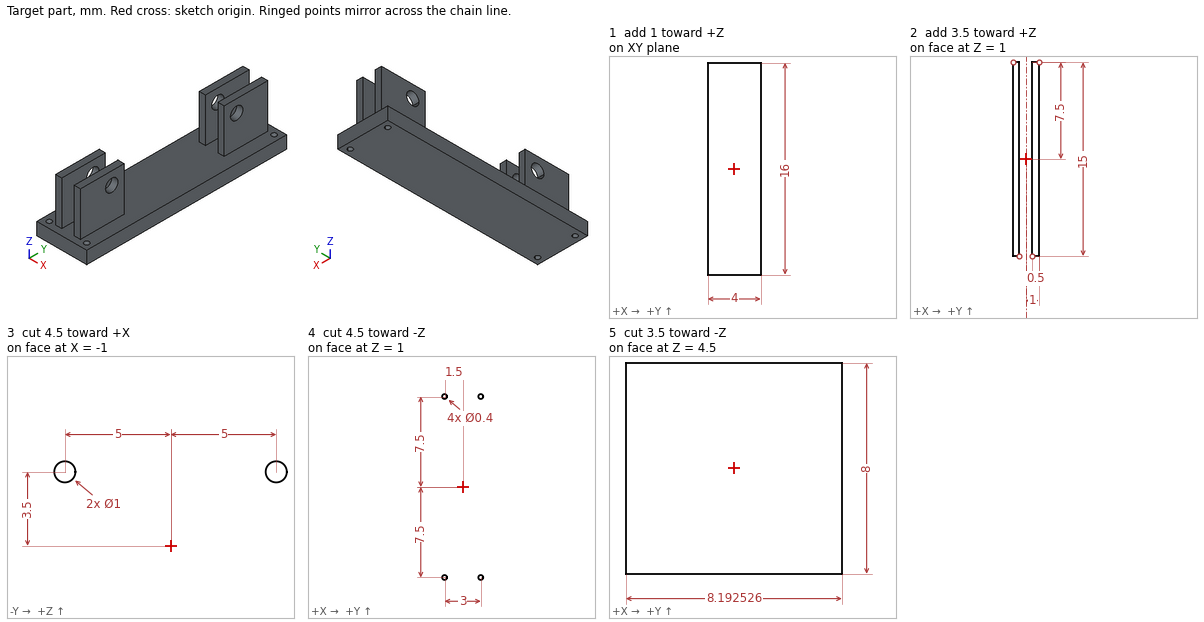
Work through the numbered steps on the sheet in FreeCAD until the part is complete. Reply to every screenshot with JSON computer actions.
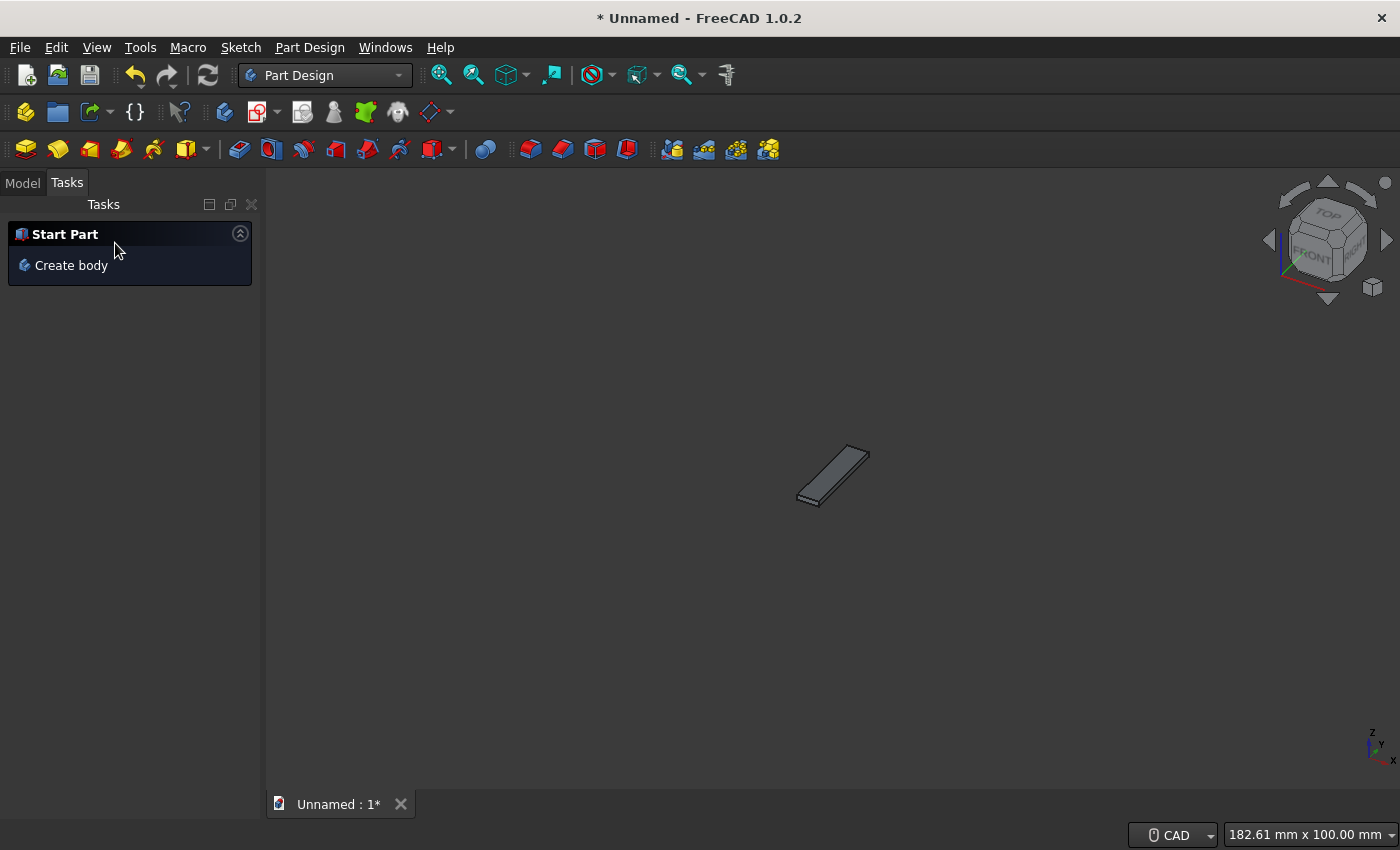
{"action": "key", "text": "v f"}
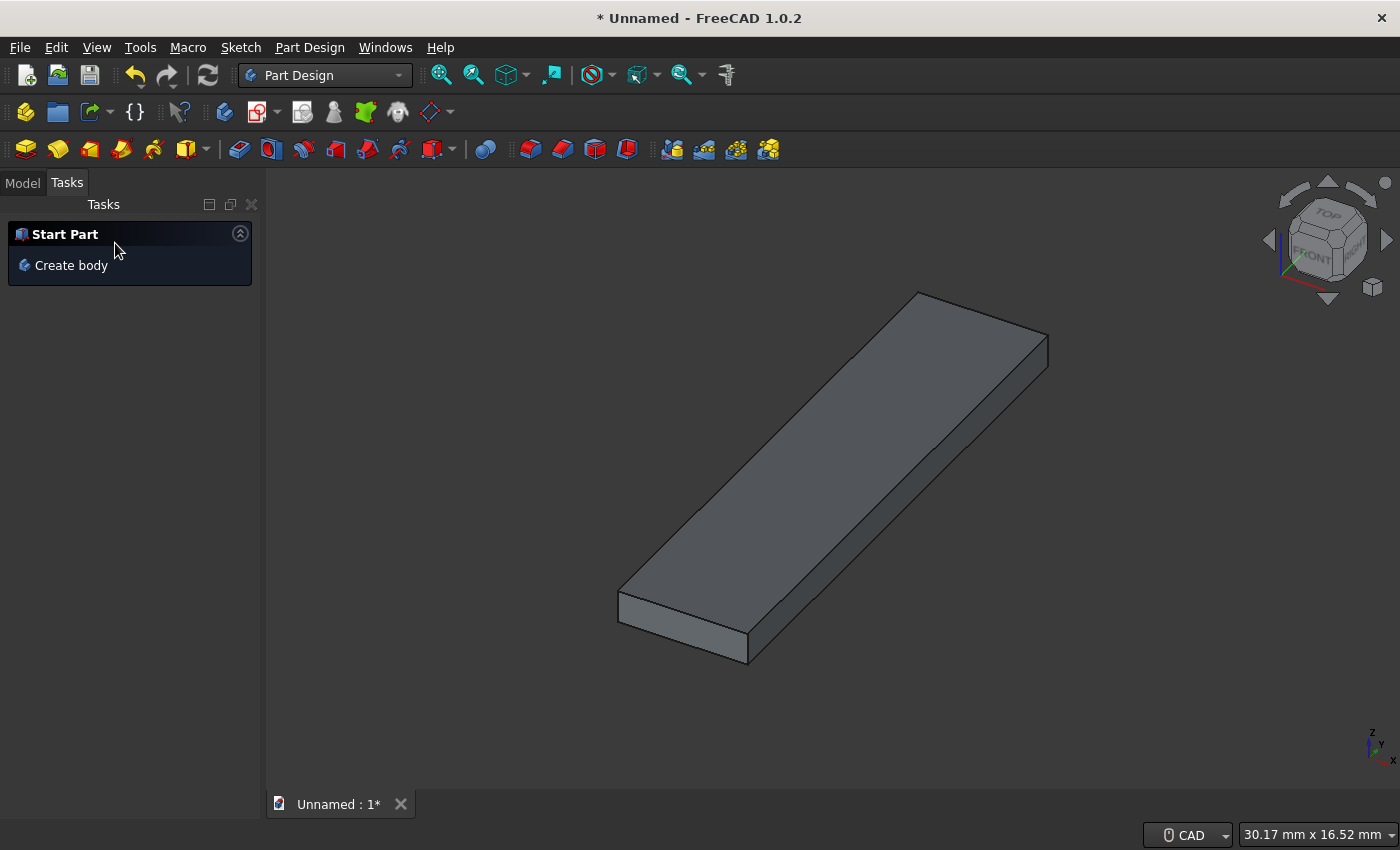
{"action": "left_click", "coordinate": [919, 377]}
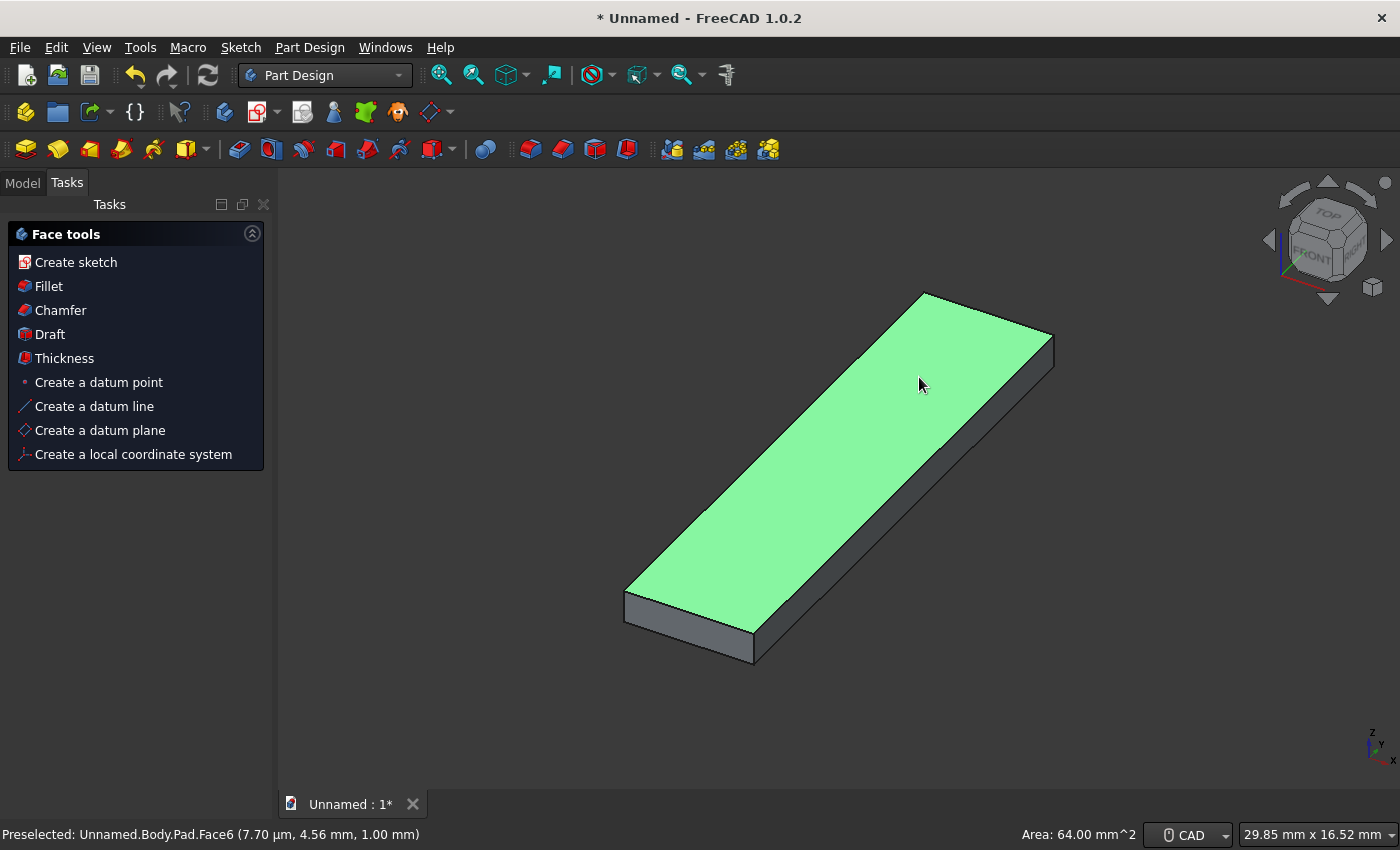
{"action": "left_click", "coordinate": [258, 112]}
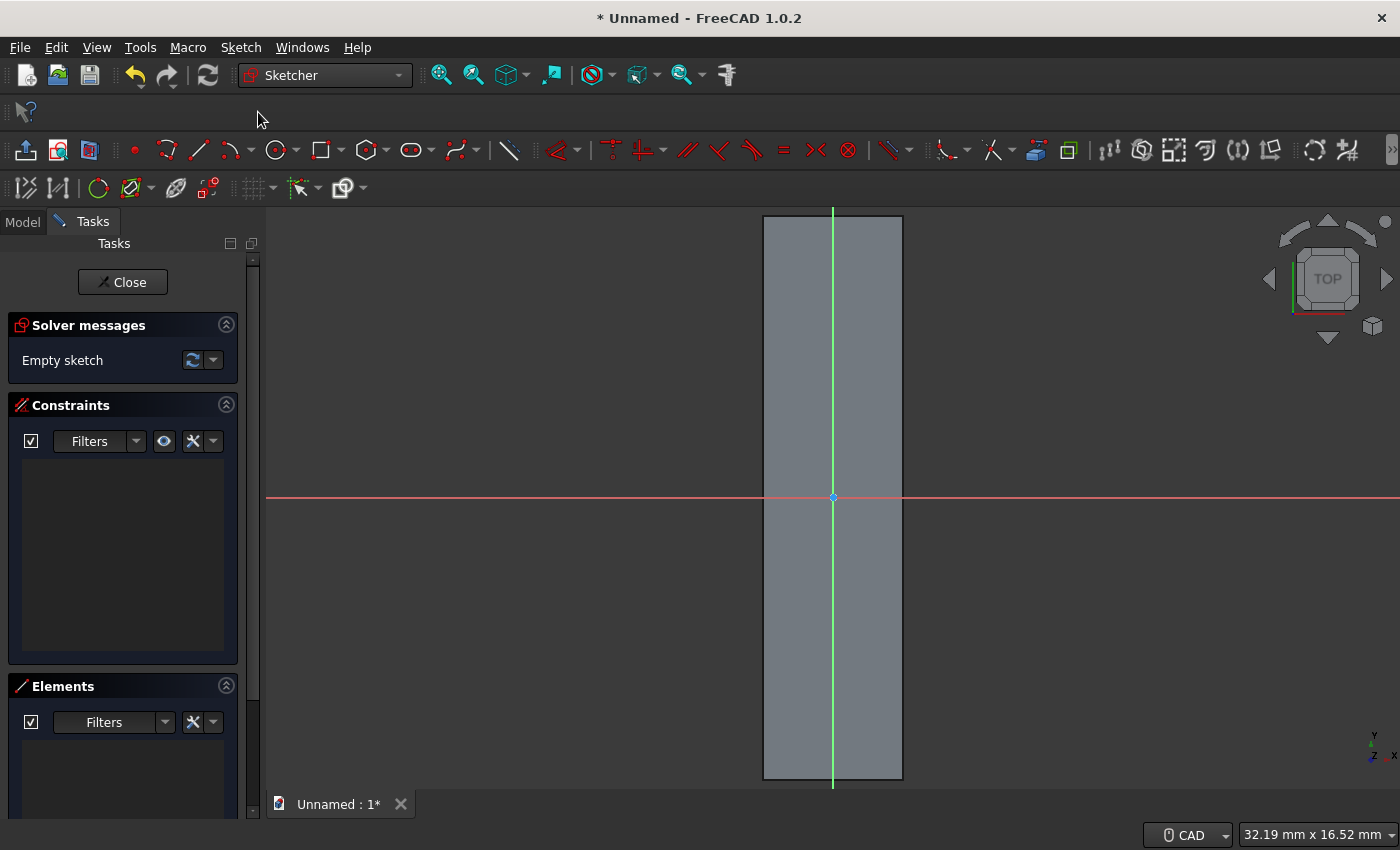
{"action": "scroll", "coordinate": [625, 498], "scroll_direction": "down", "scroll_amount": 2}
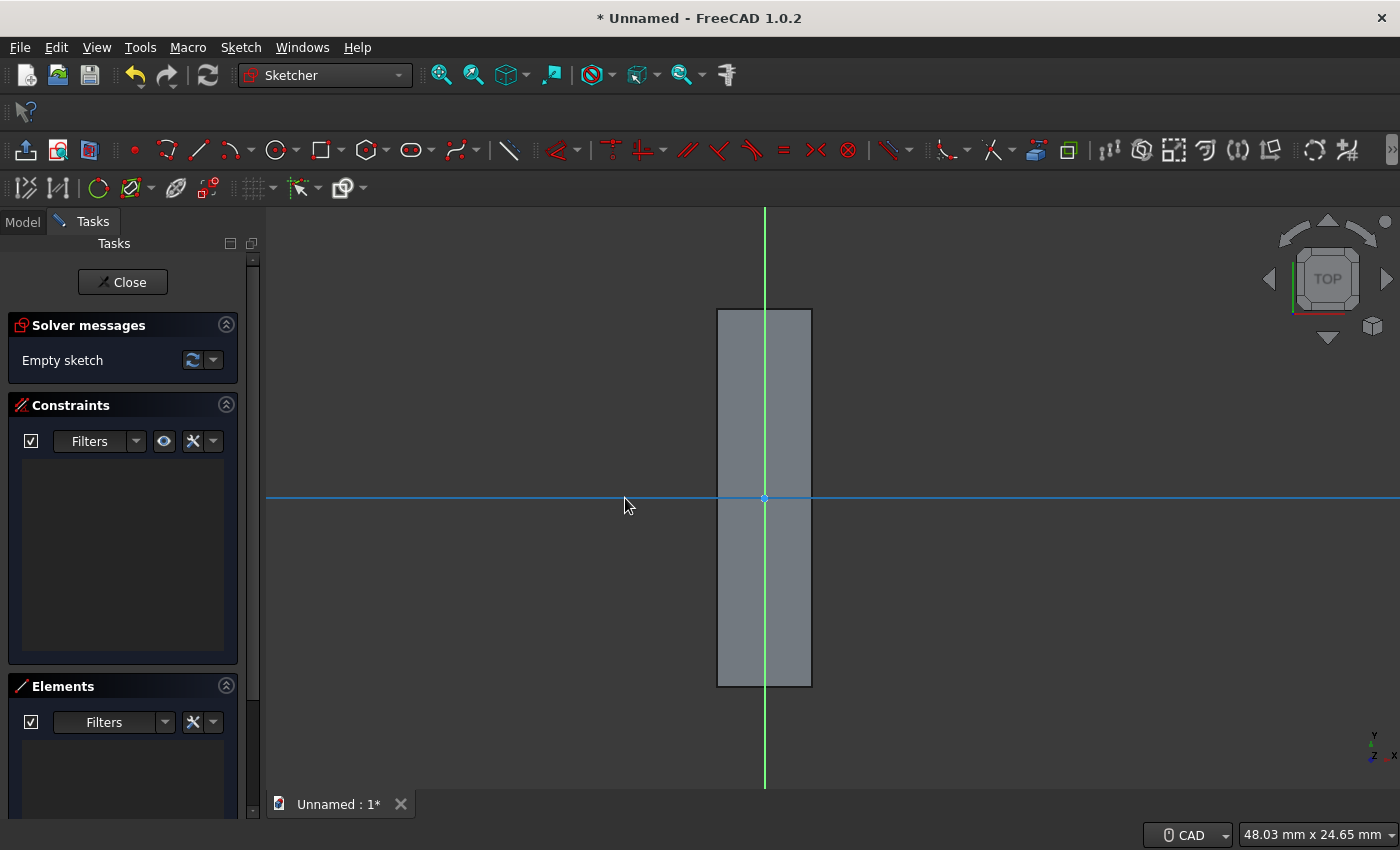
{"action": "left_click", "coordinate": [322, 150]}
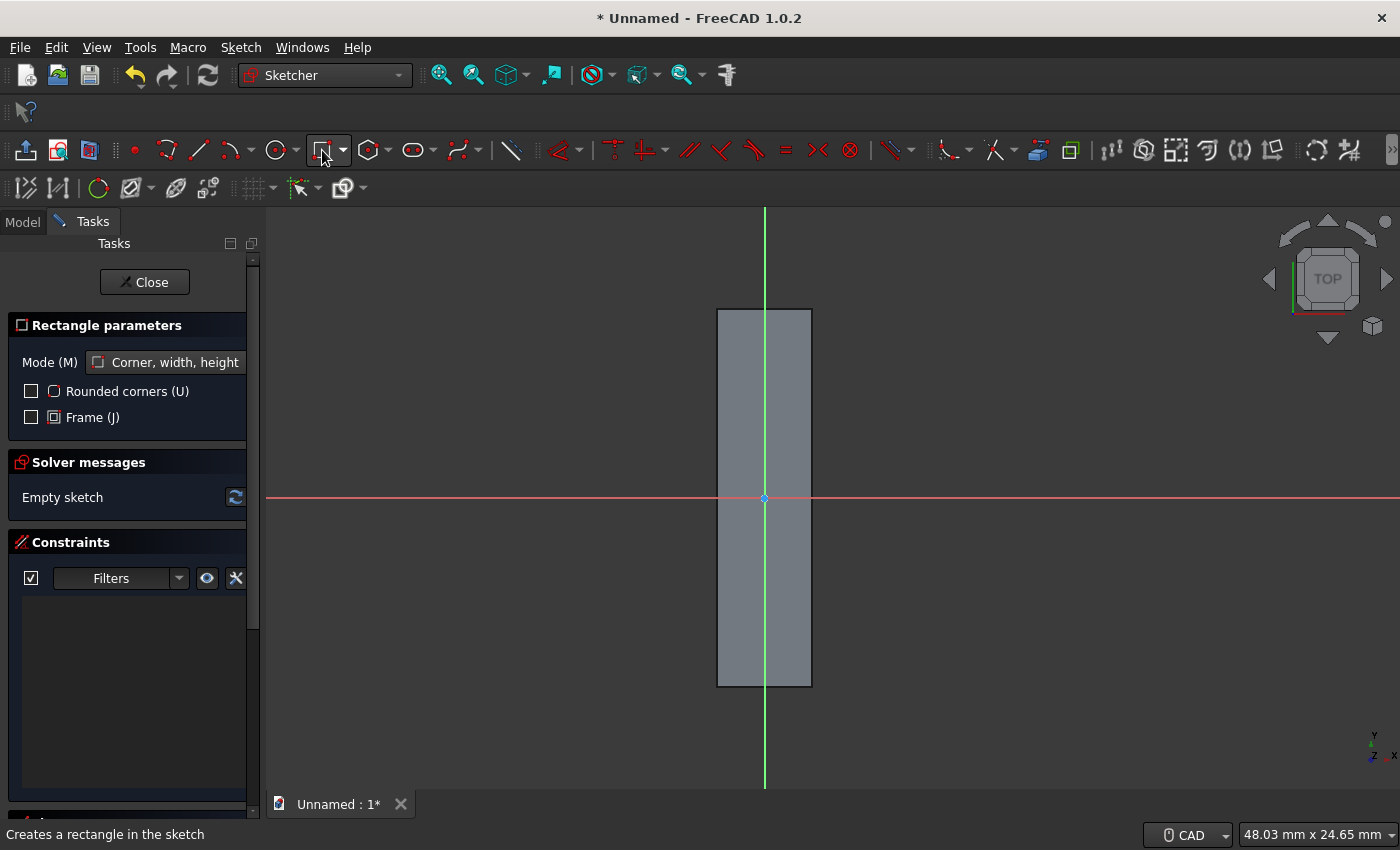
{"action": "scroll", "coordinate": [776, 321], "scroll_direction": "up", "scroll_amount": 2}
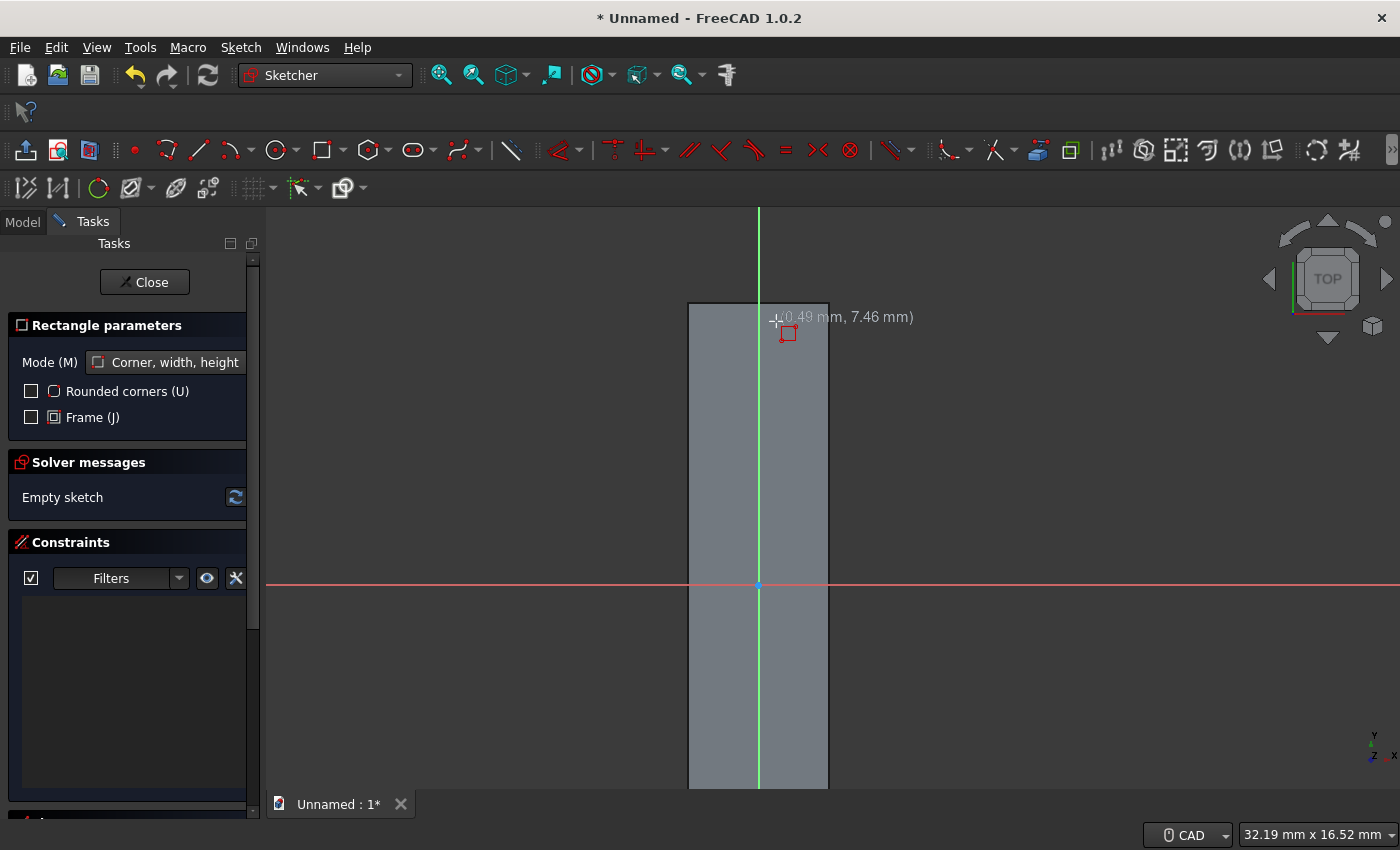
{"action": "left_click", "coordinate": [776, 321]}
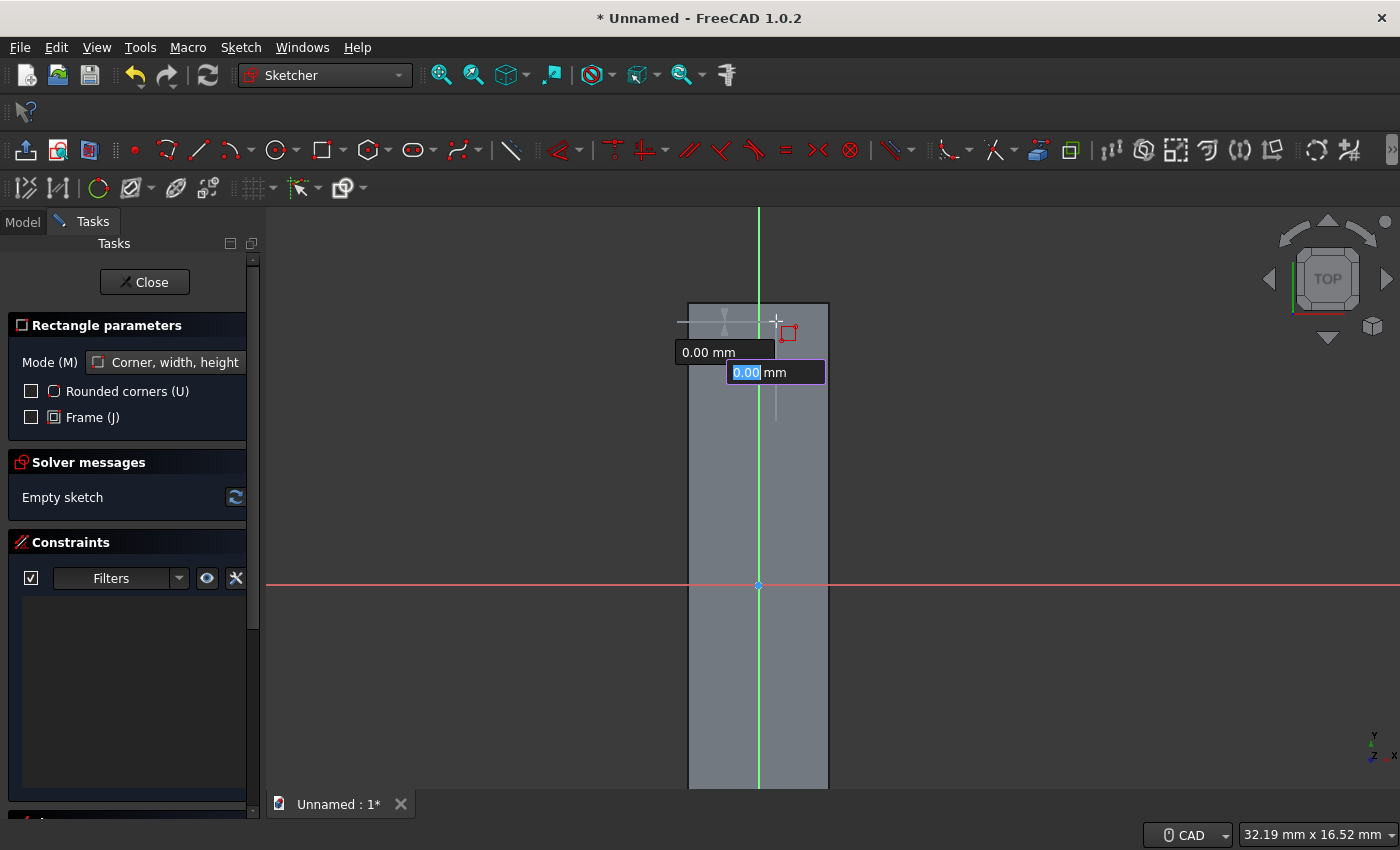
{"action": "scroll", "coordinate": [776, 321], "scroll_direction": "down", "scroll_amount": 2}